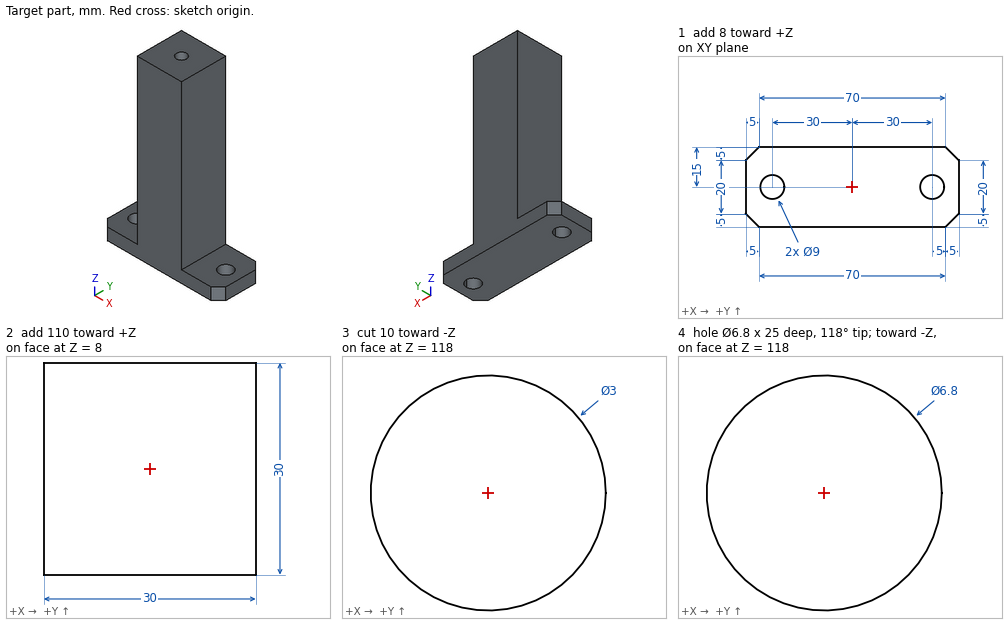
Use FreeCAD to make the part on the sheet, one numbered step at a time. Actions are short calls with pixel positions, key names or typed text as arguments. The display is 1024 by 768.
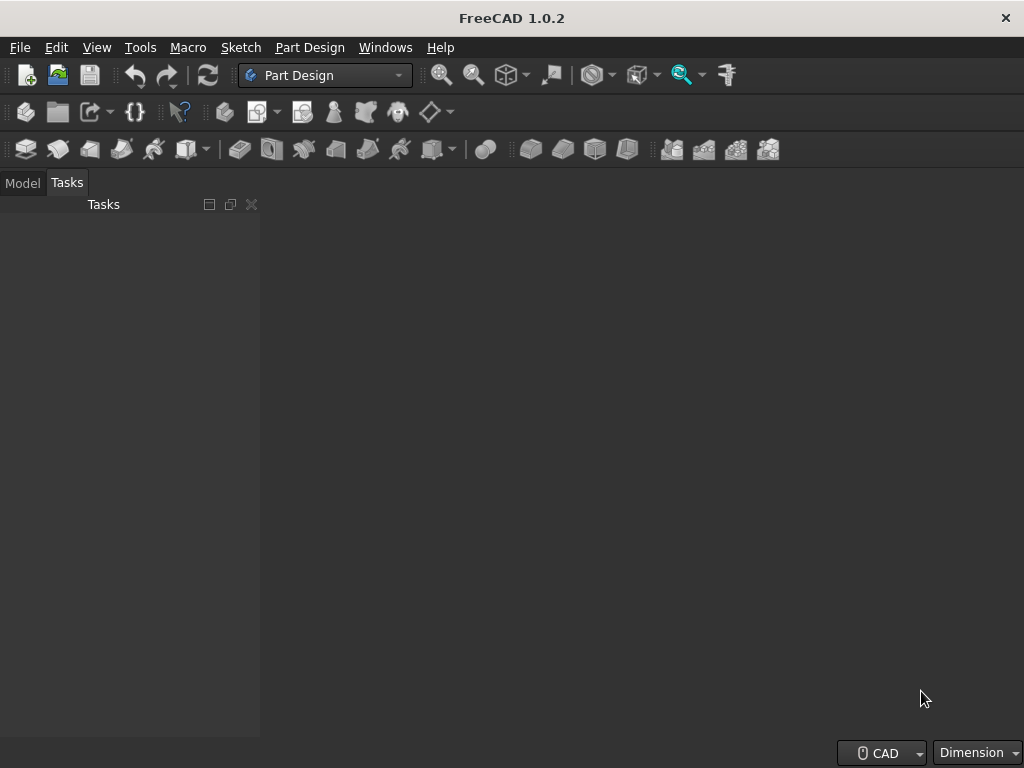
click(26, 76)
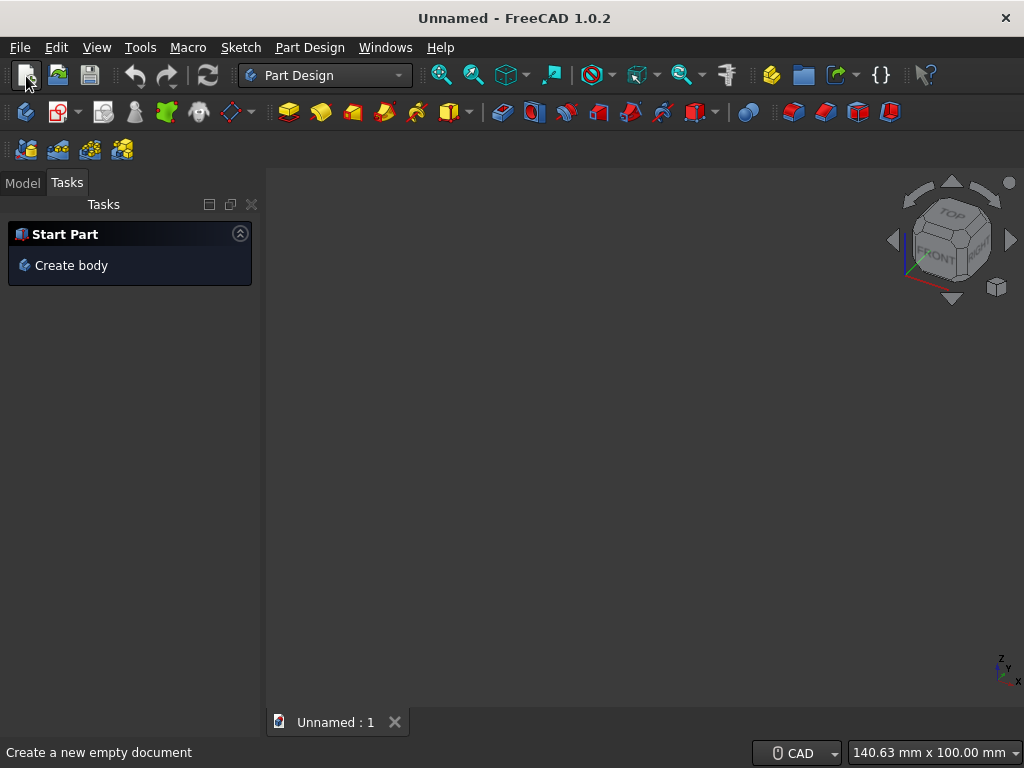
click(58, 112)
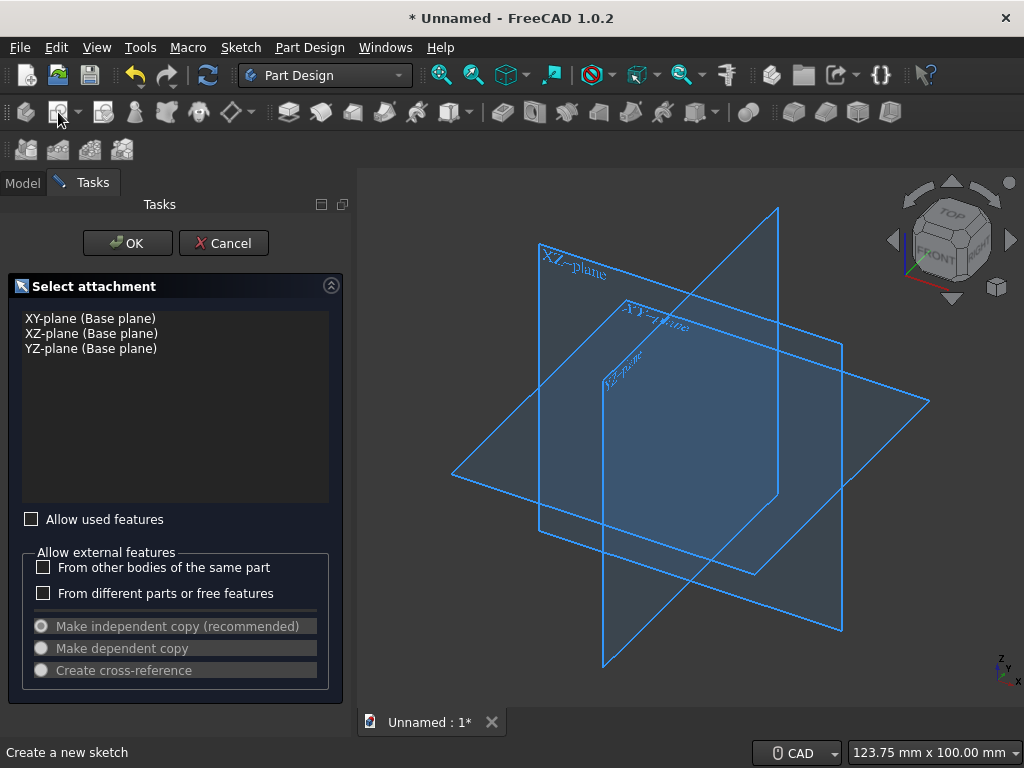
click(82, 318)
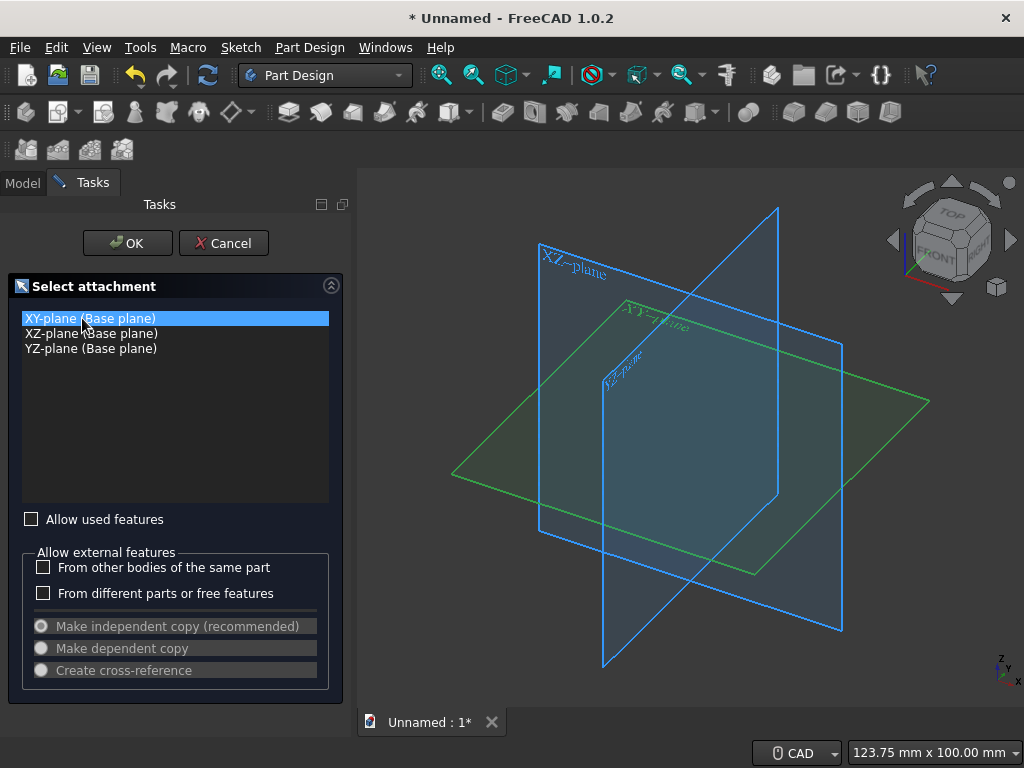
click(128, 243)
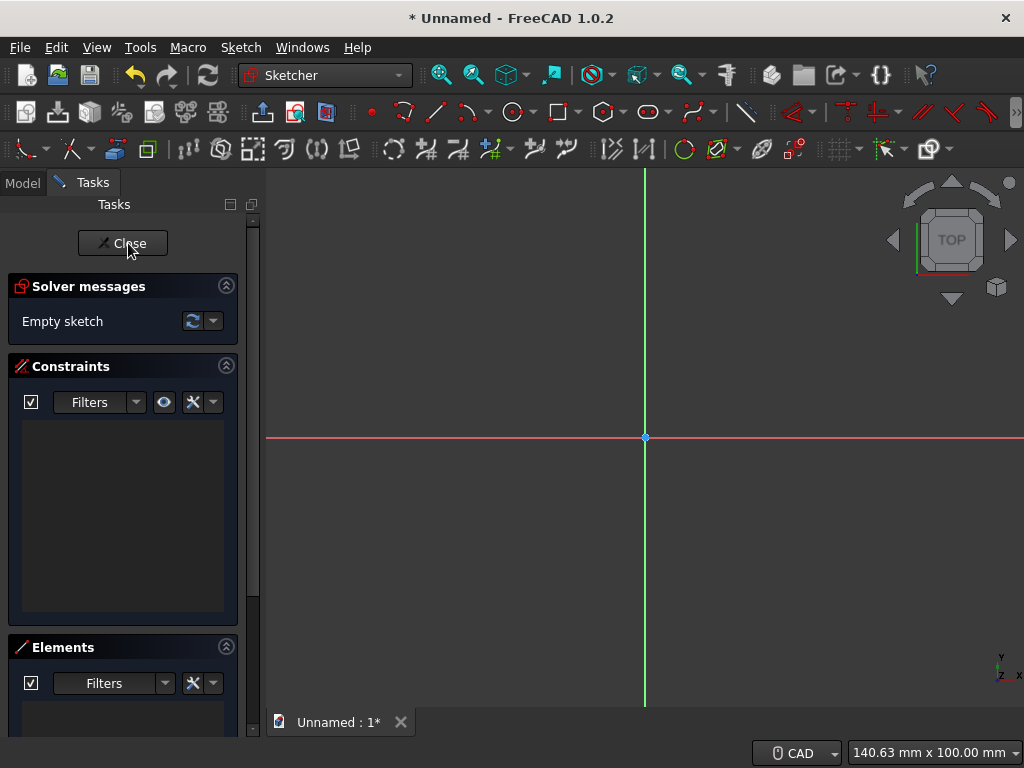
scroll(294, 437, down, 1)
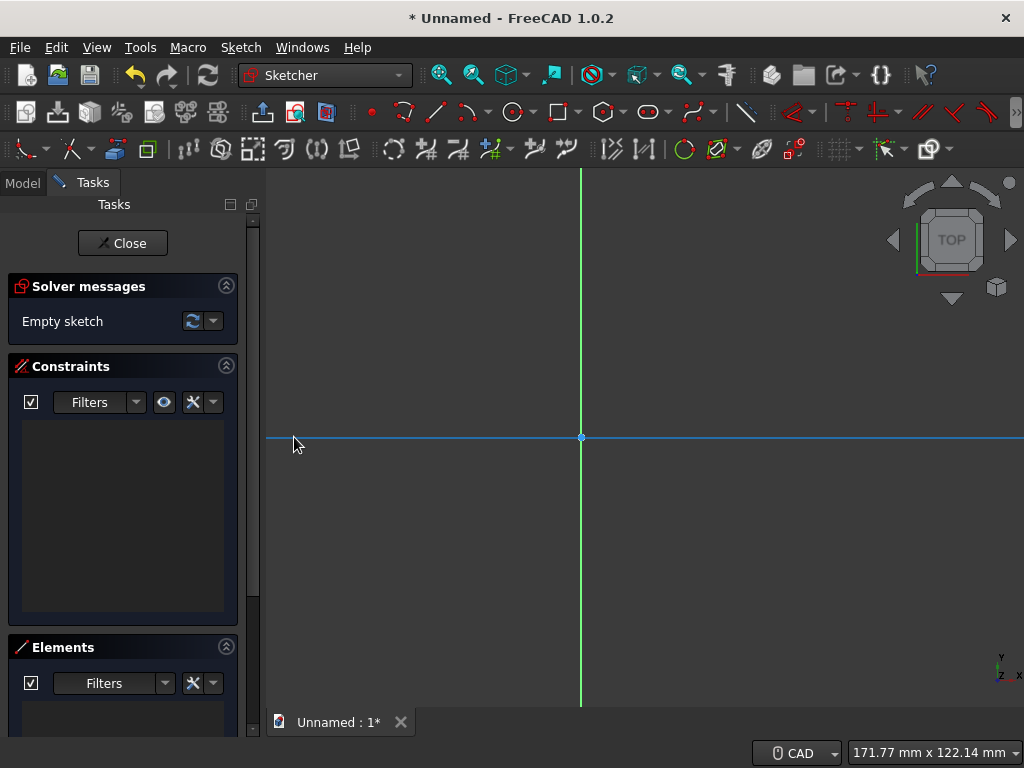
click(404, 112)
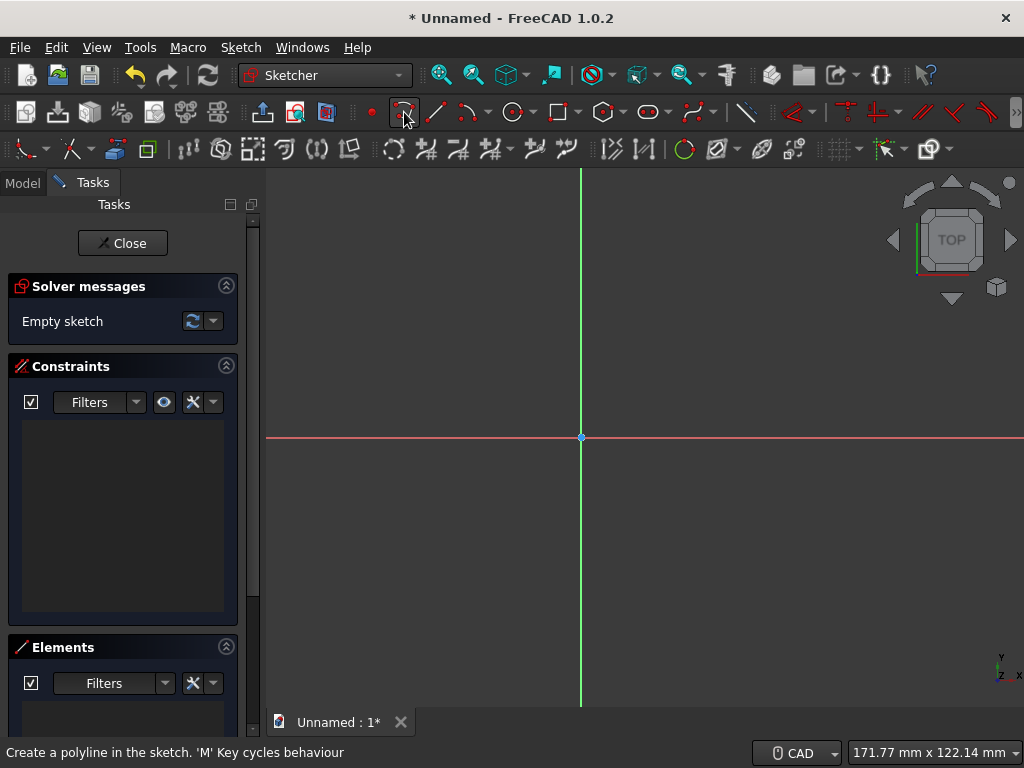
click(427, 371)
click(405, 393)
click(405, 482)
click(427, 504)
click(736, 504)
click(758, 482)
click(758, 393)
click(736, 371)
click(427, 372)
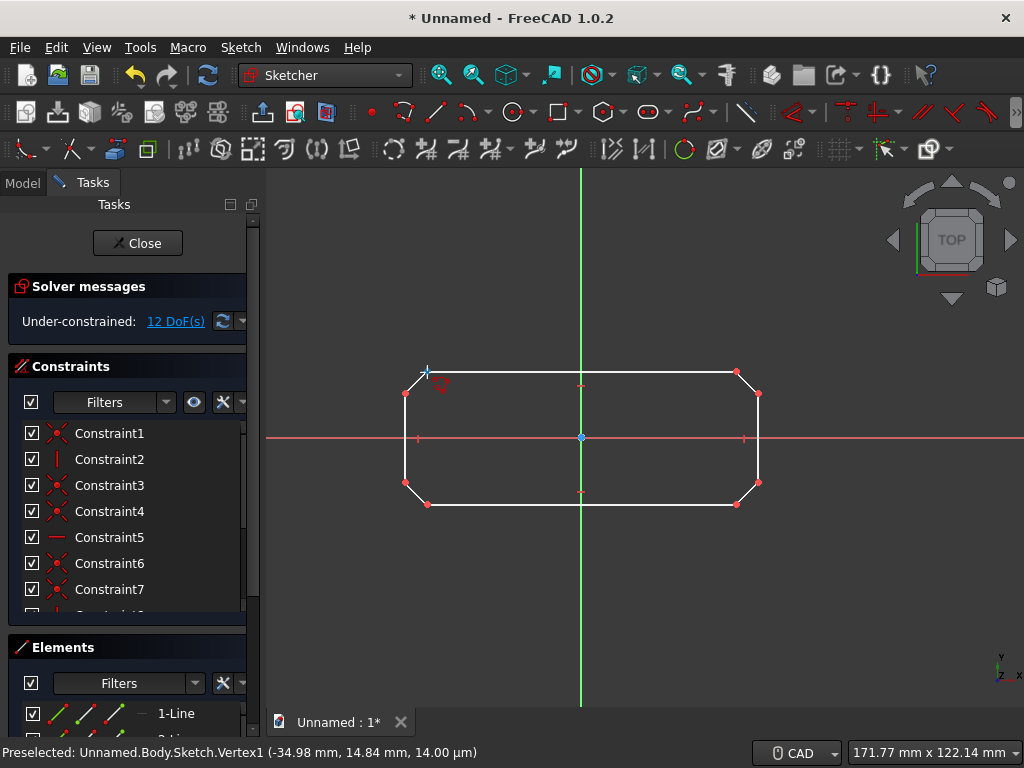
click(514, 112)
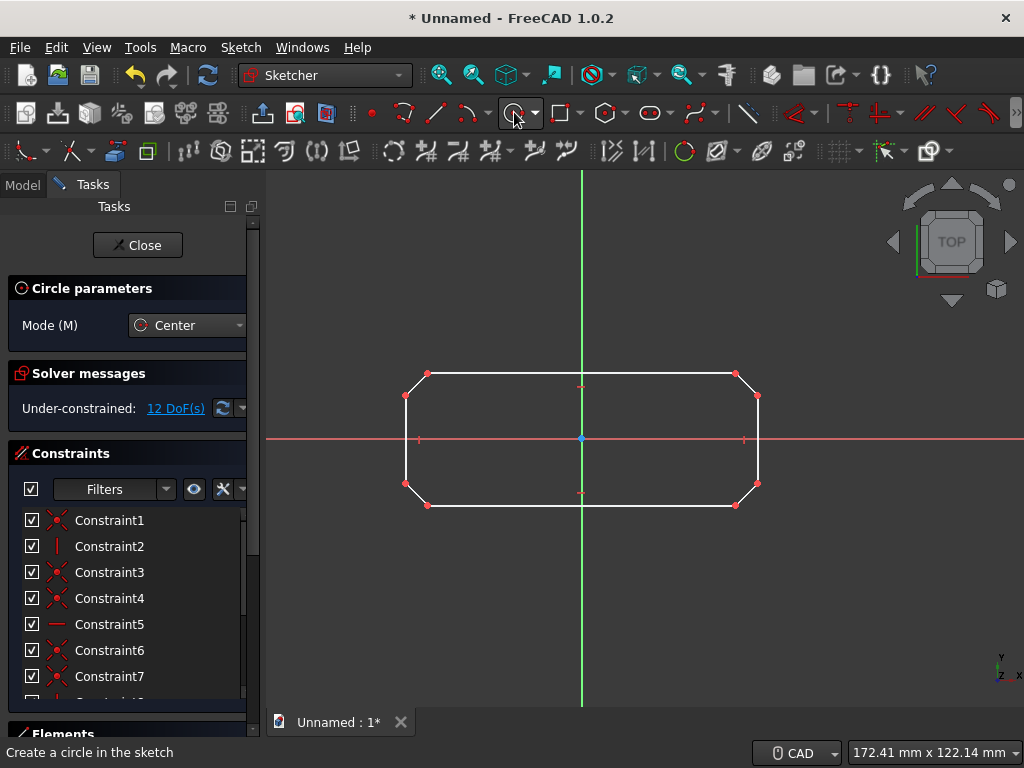
click(714, 438)
click(720, 420)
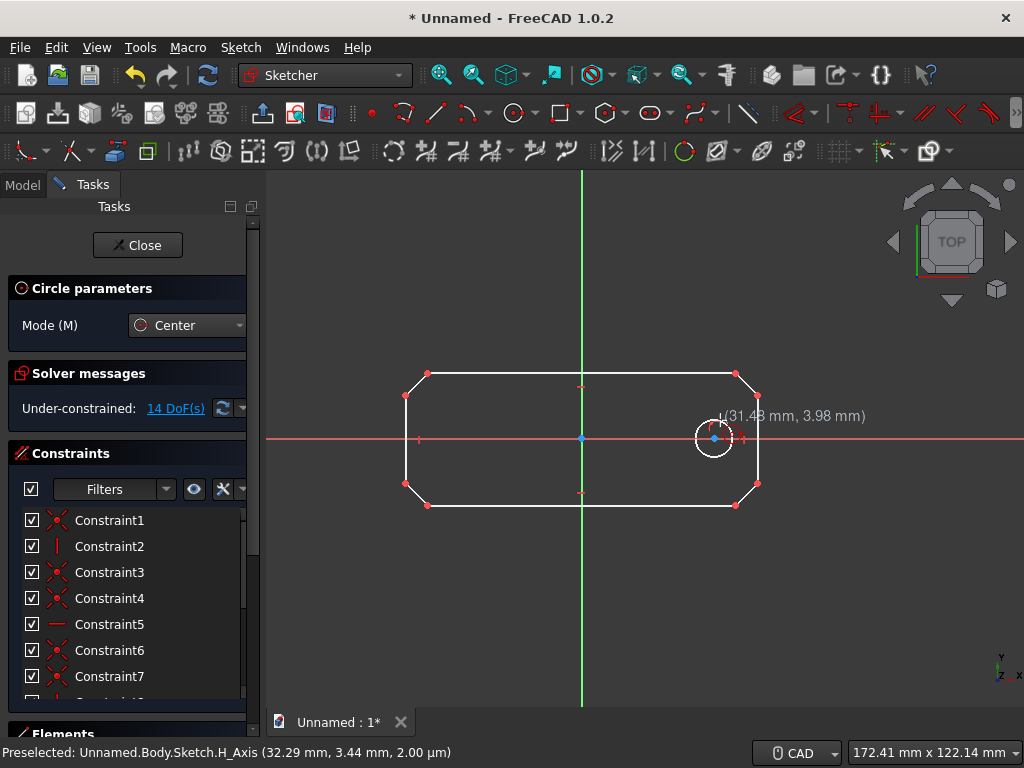
click(450, 438)
click(456, 420)
key(Escape)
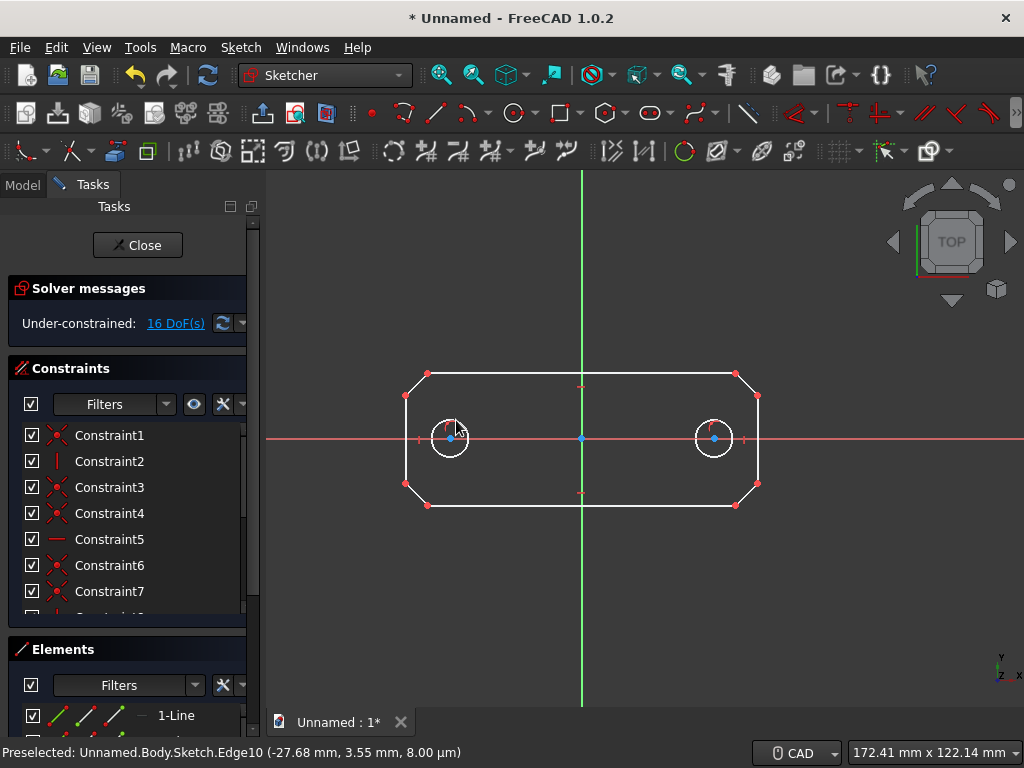
click(727, 425)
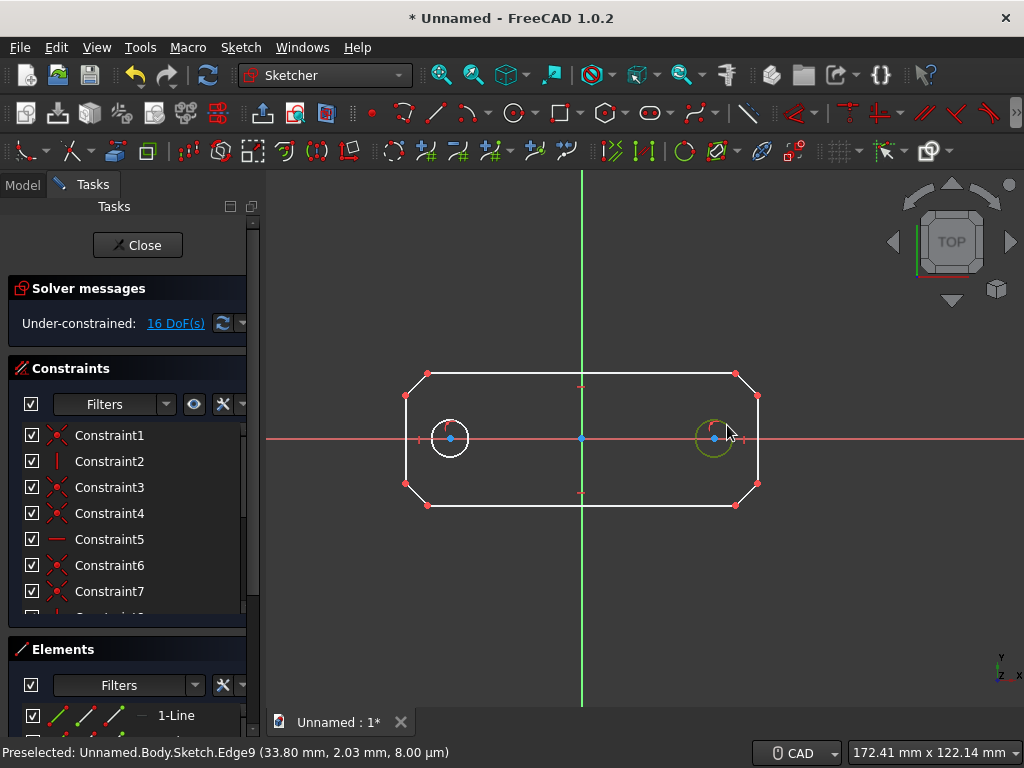
click(463, 425)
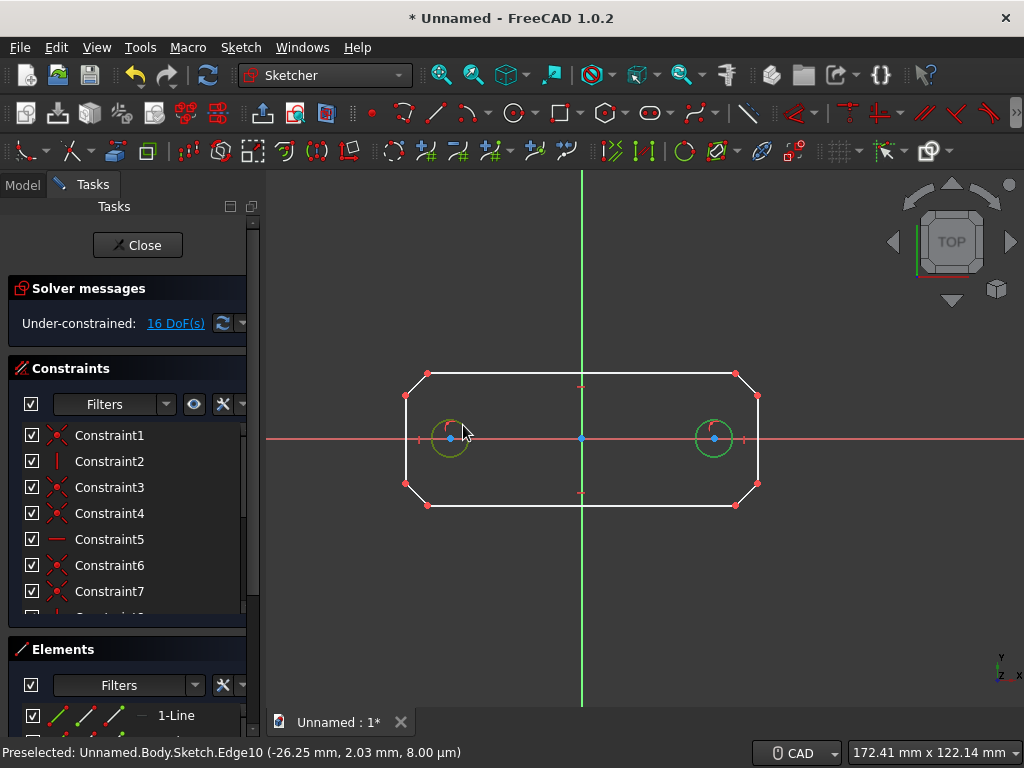
key(e)